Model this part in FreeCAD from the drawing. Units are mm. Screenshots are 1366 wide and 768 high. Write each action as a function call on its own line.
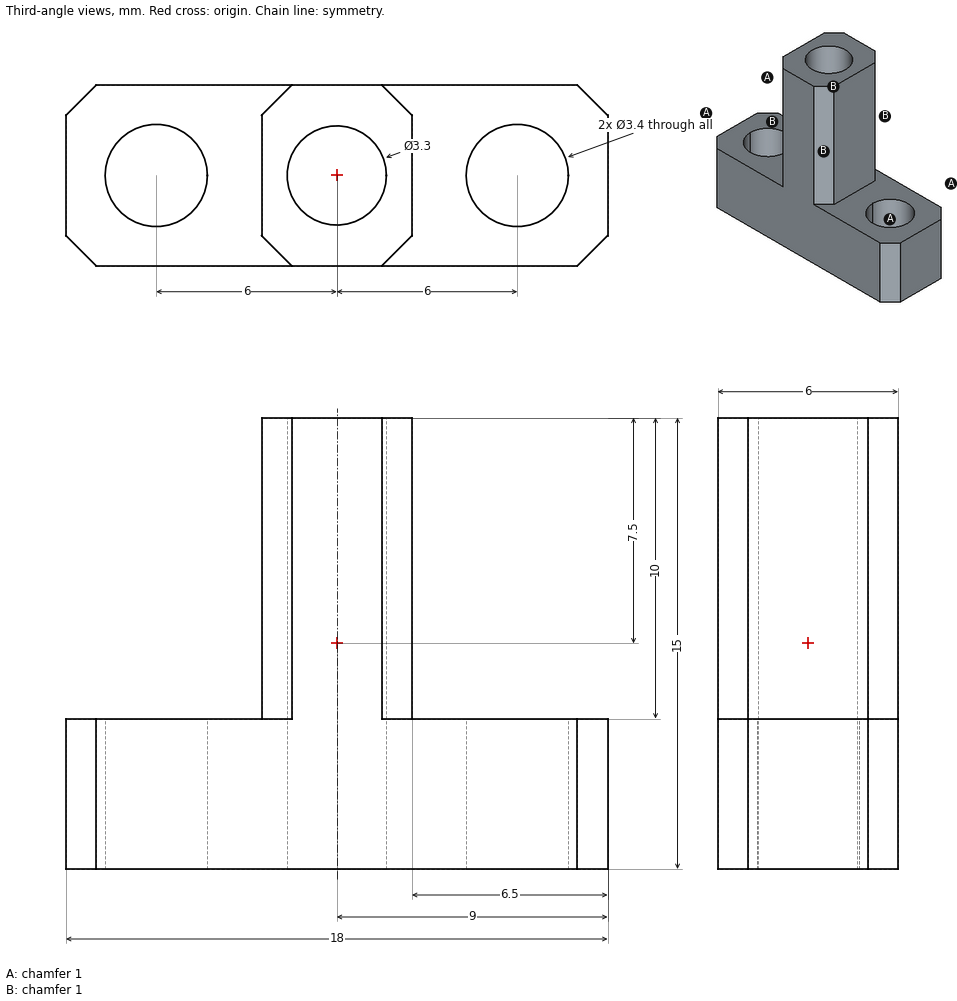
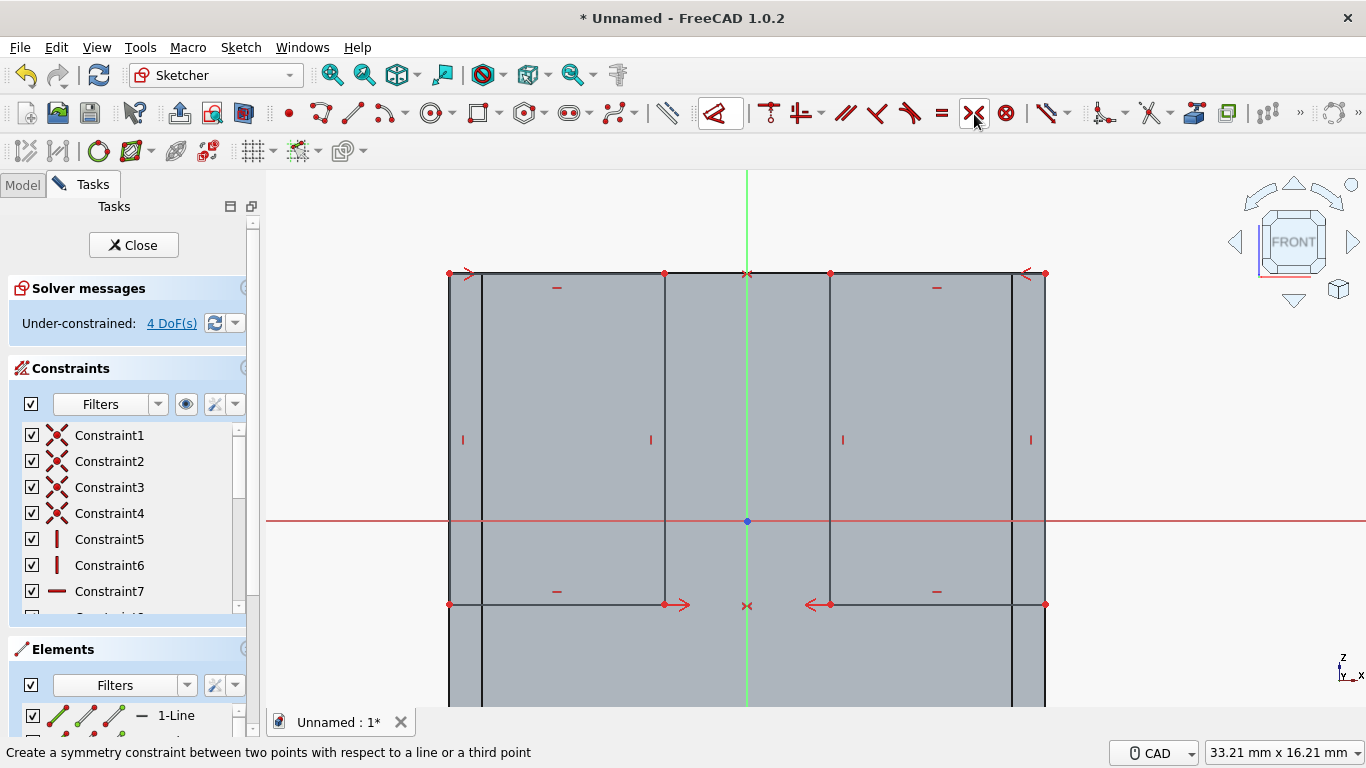
click(830, 373)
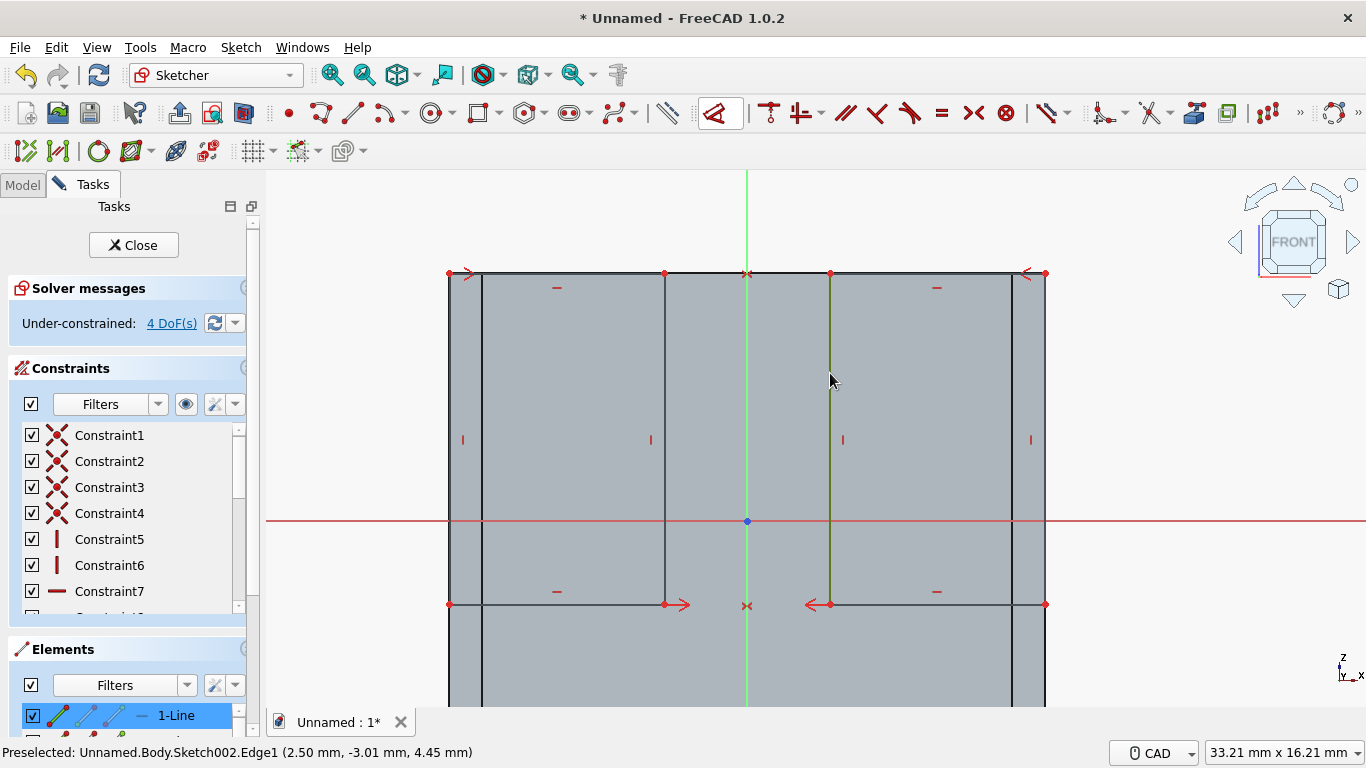
click(738, 114)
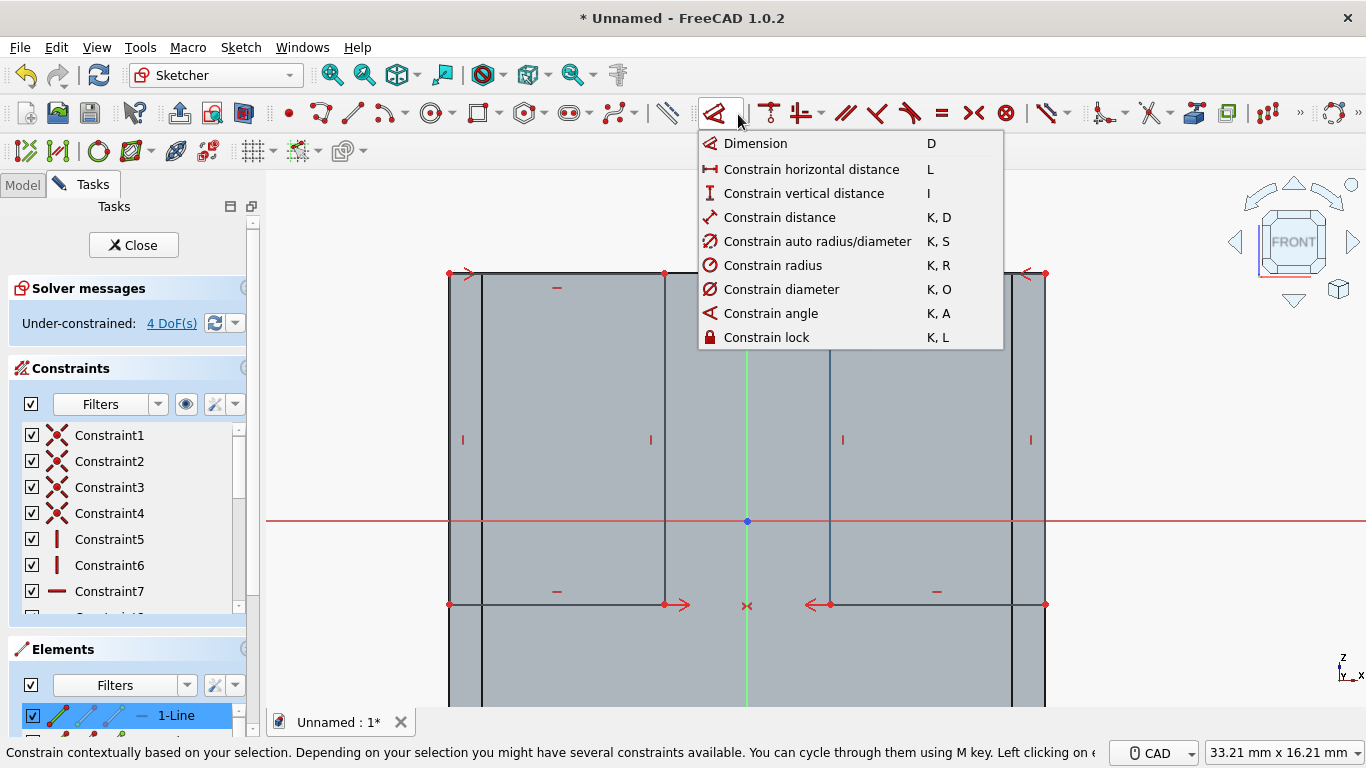
click(851, 193)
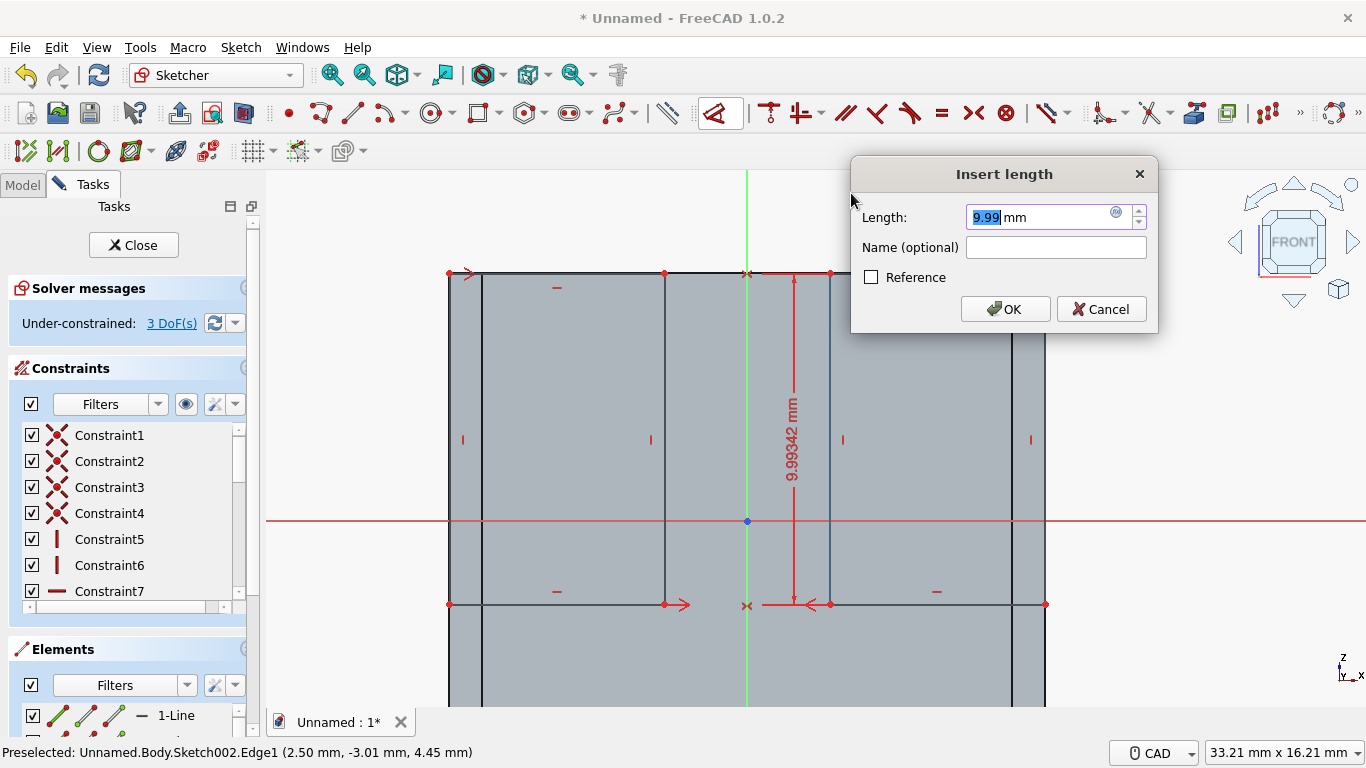
text(10)
key(Return)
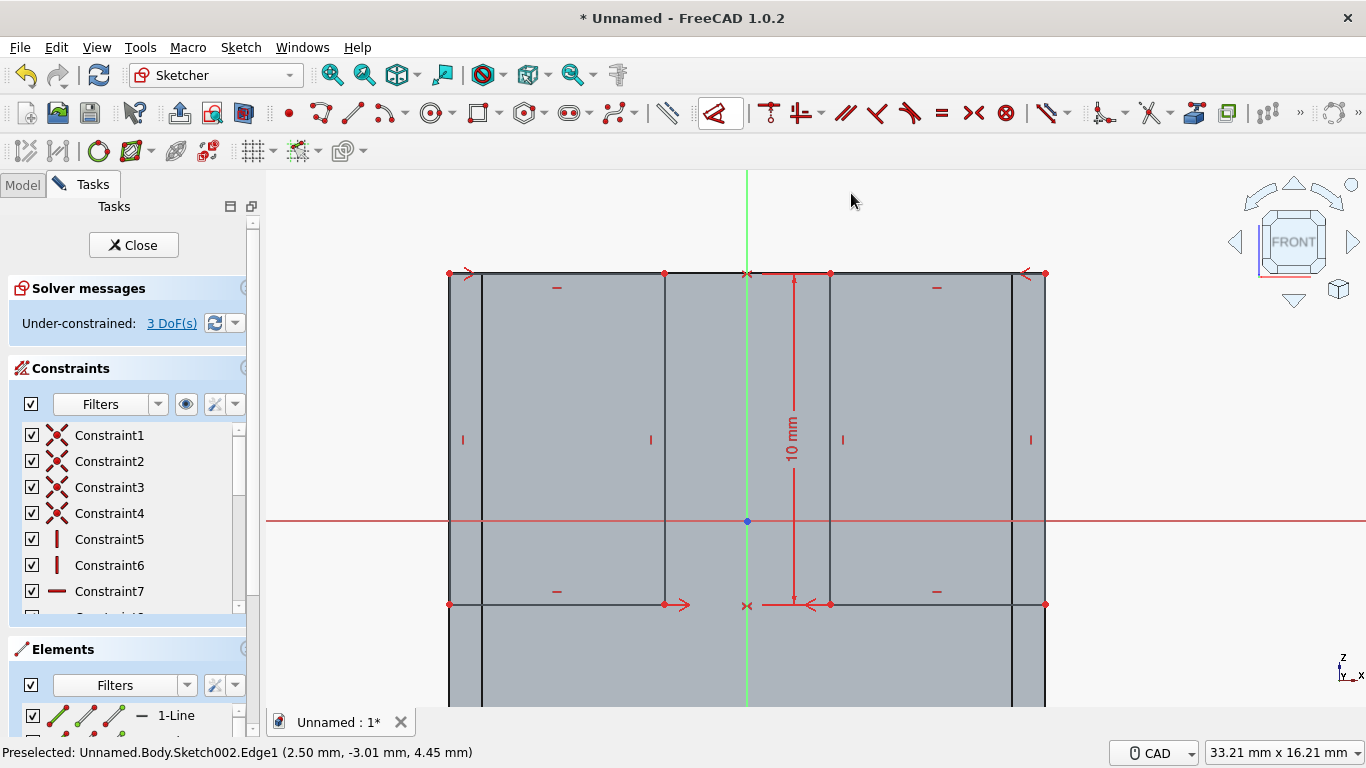
click(1045, 605)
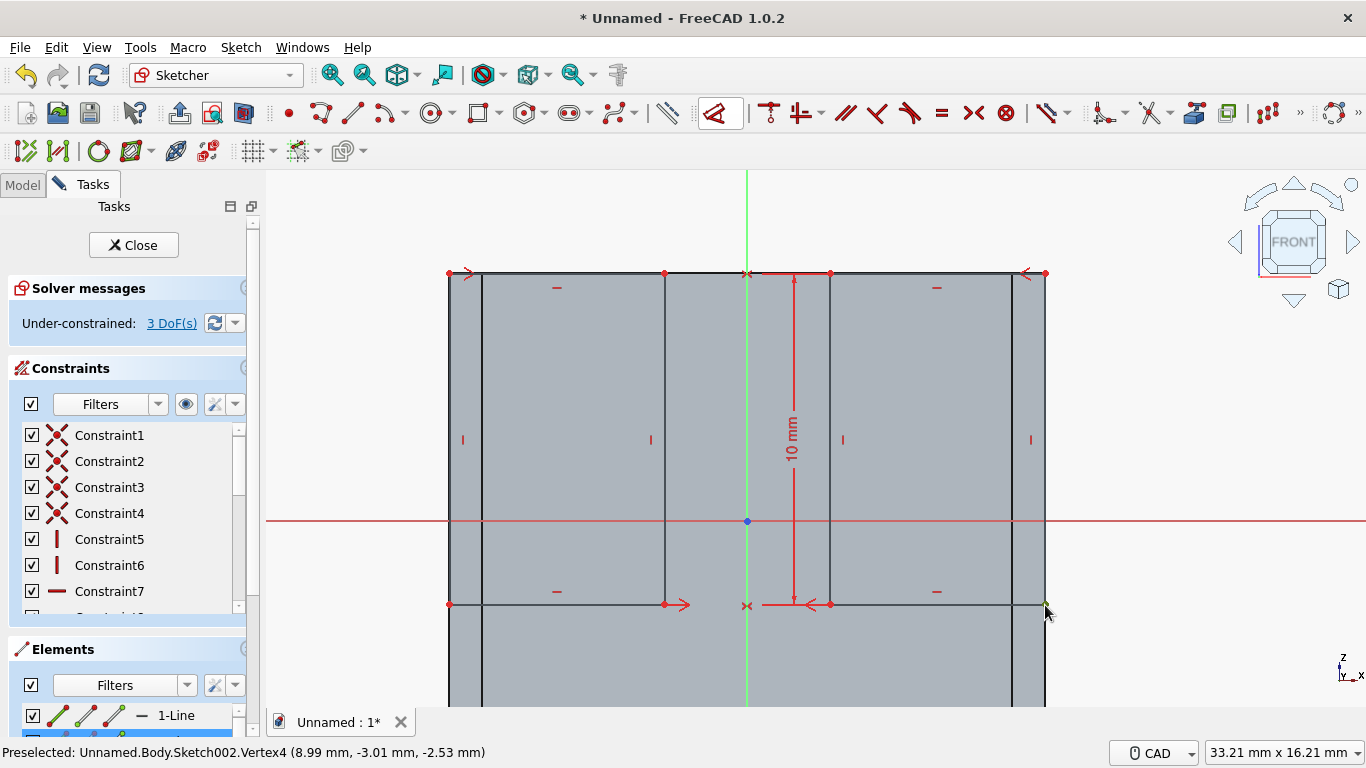
click(738, 114)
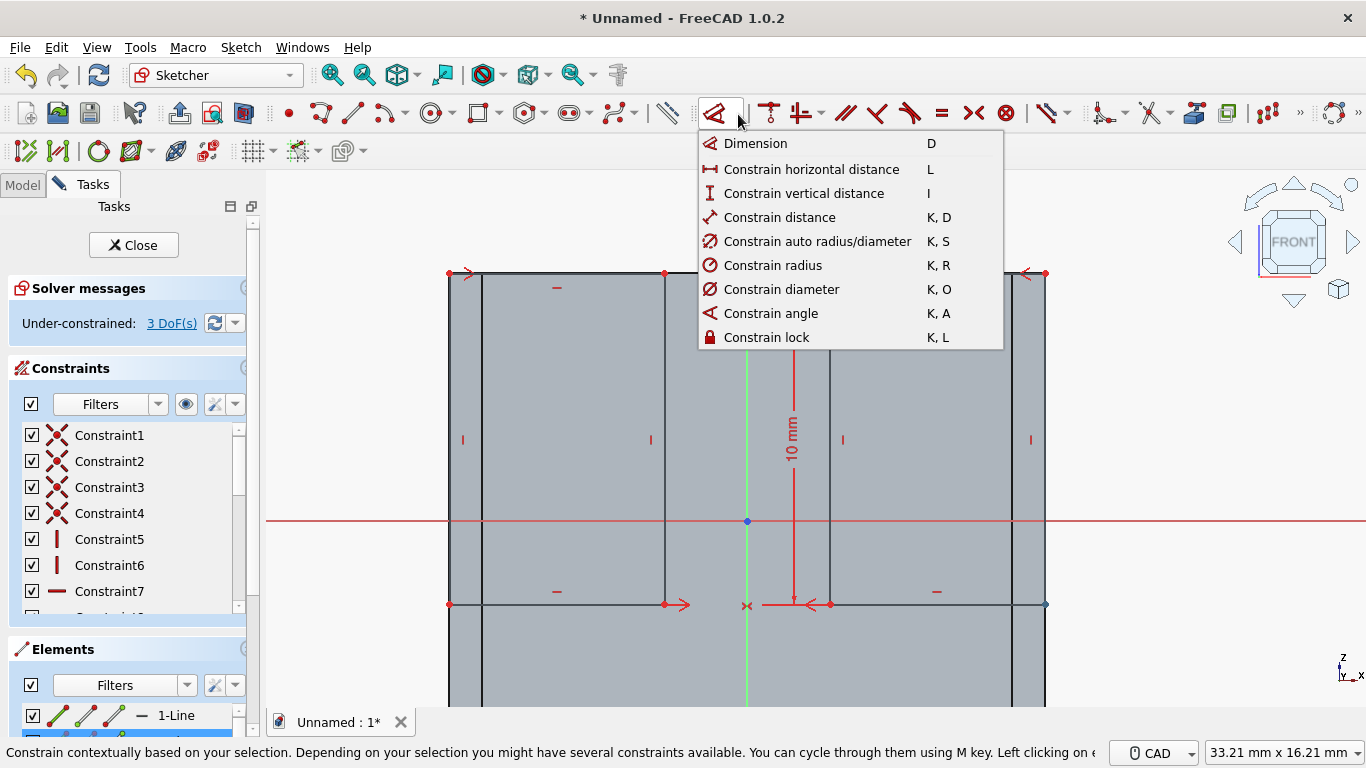
click(851, 169)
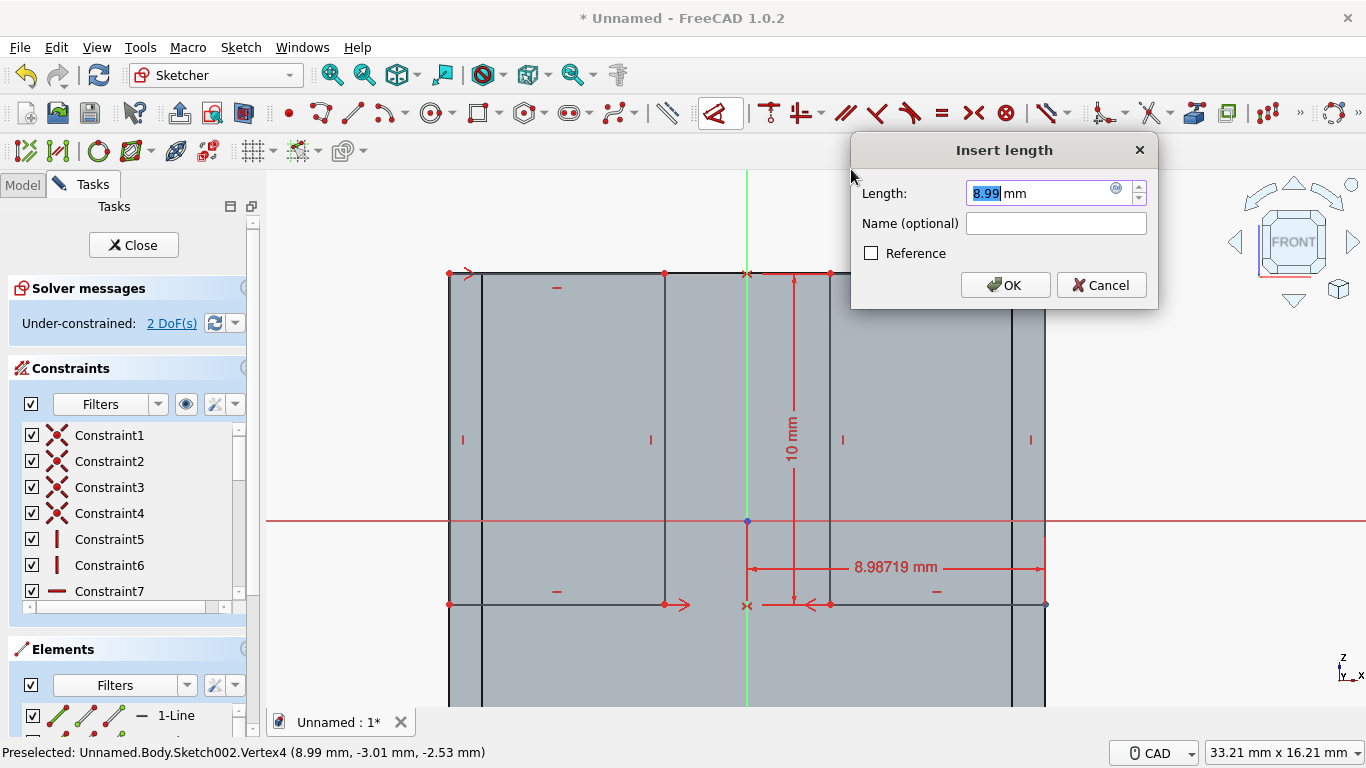
text(9)
key(Return)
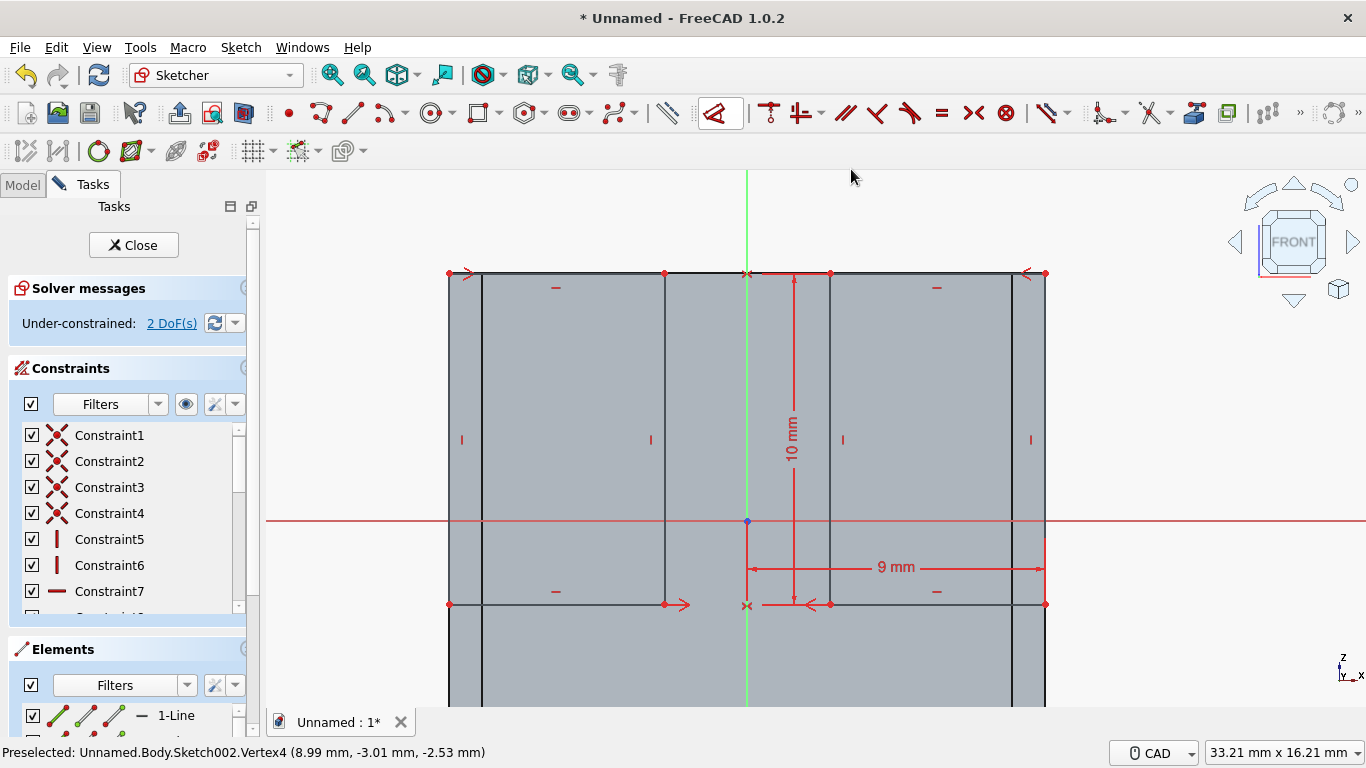
click(895, 605)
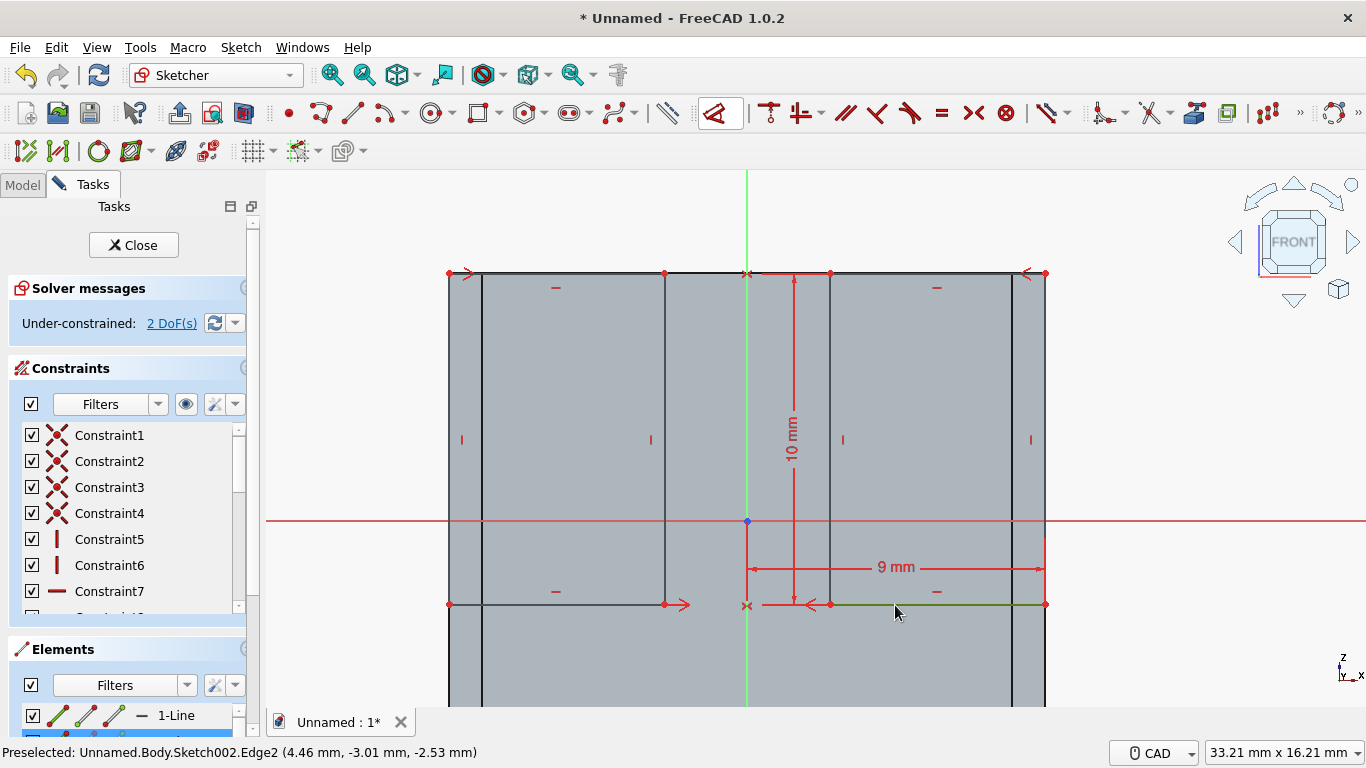
key(l)